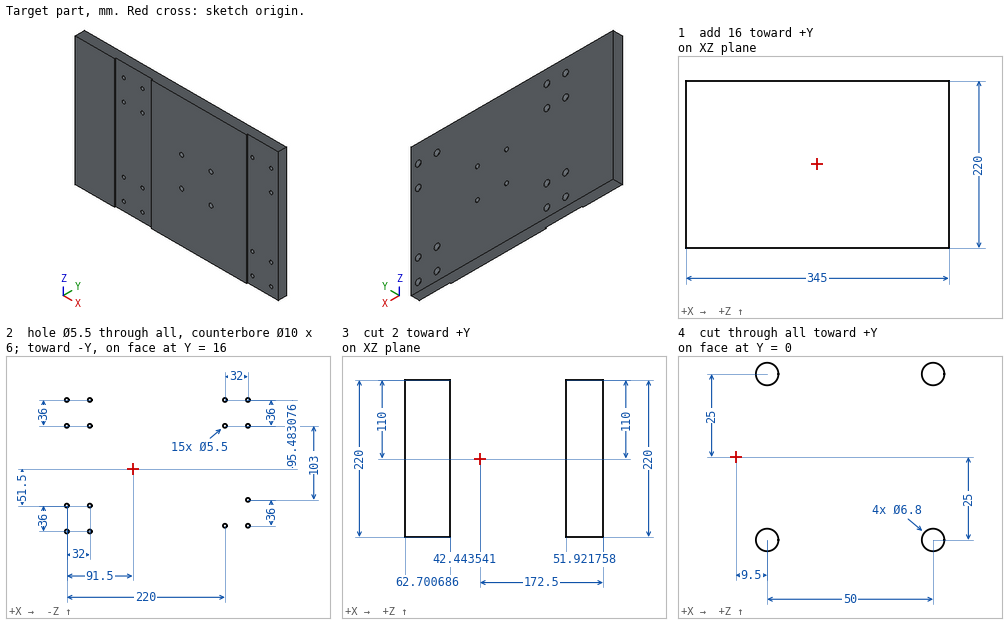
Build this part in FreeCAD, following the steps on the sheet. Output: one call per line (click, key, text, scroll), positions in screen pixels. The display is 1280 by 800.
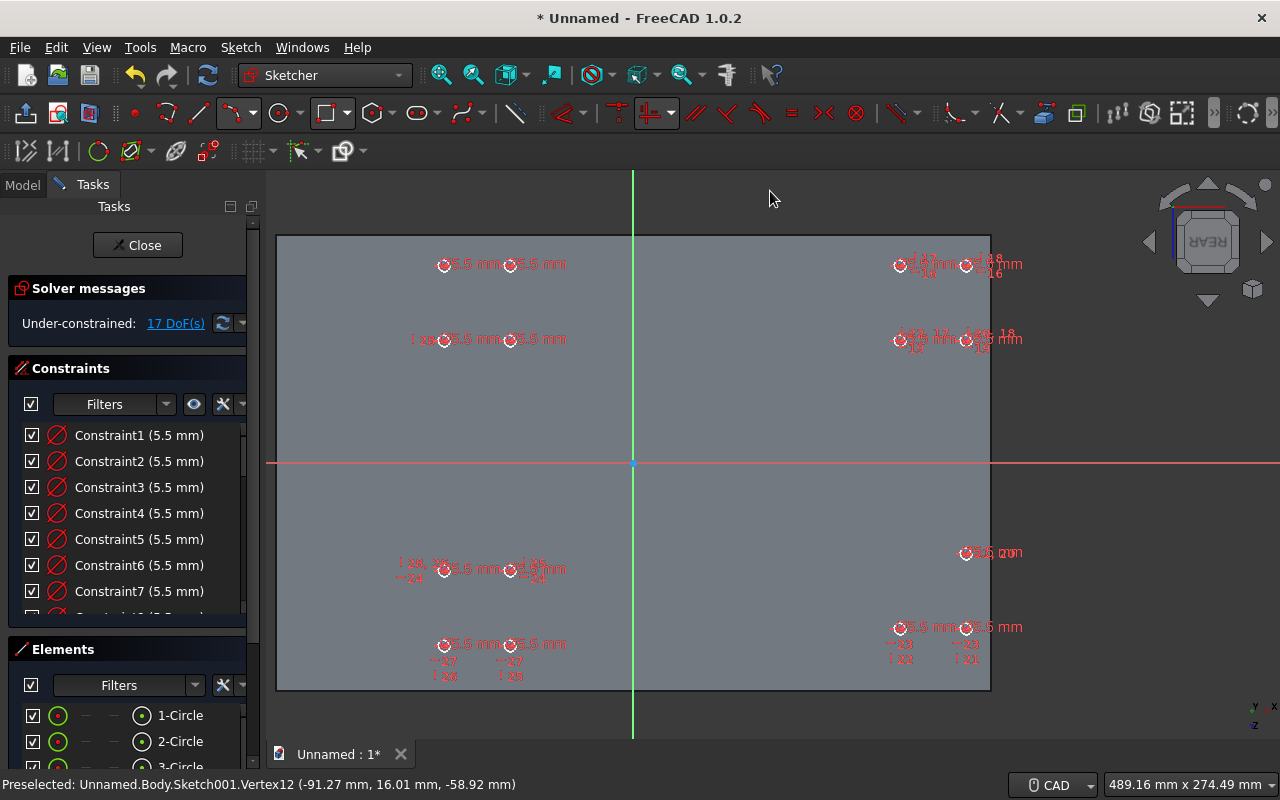
click(900, 341)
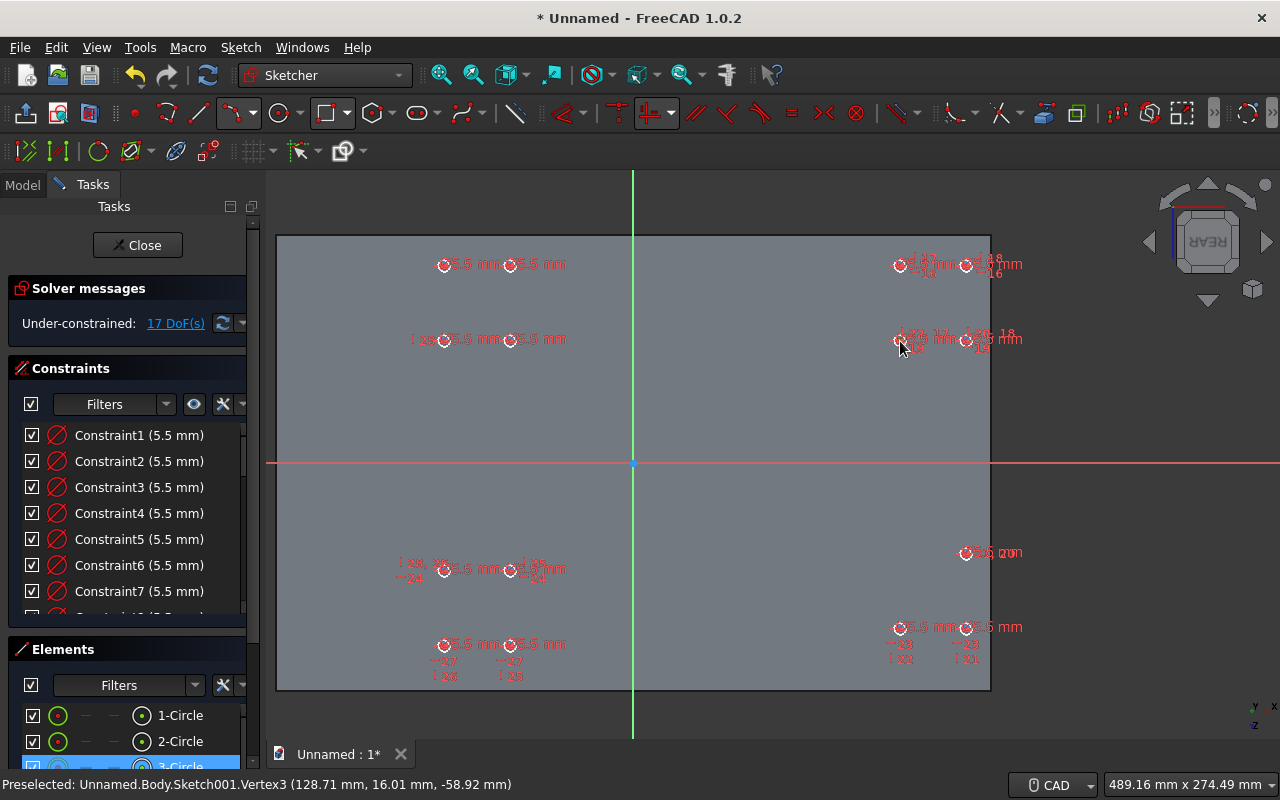
click(444, 341)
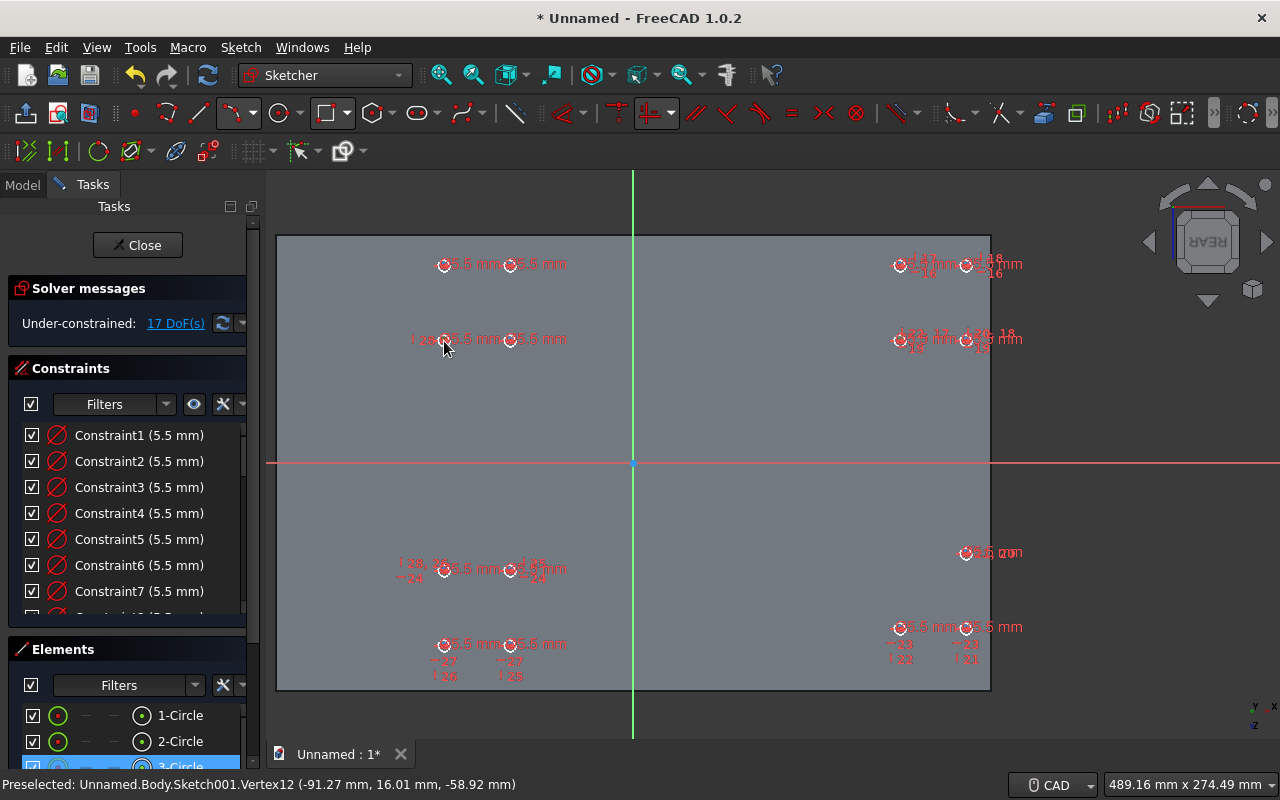
key(h)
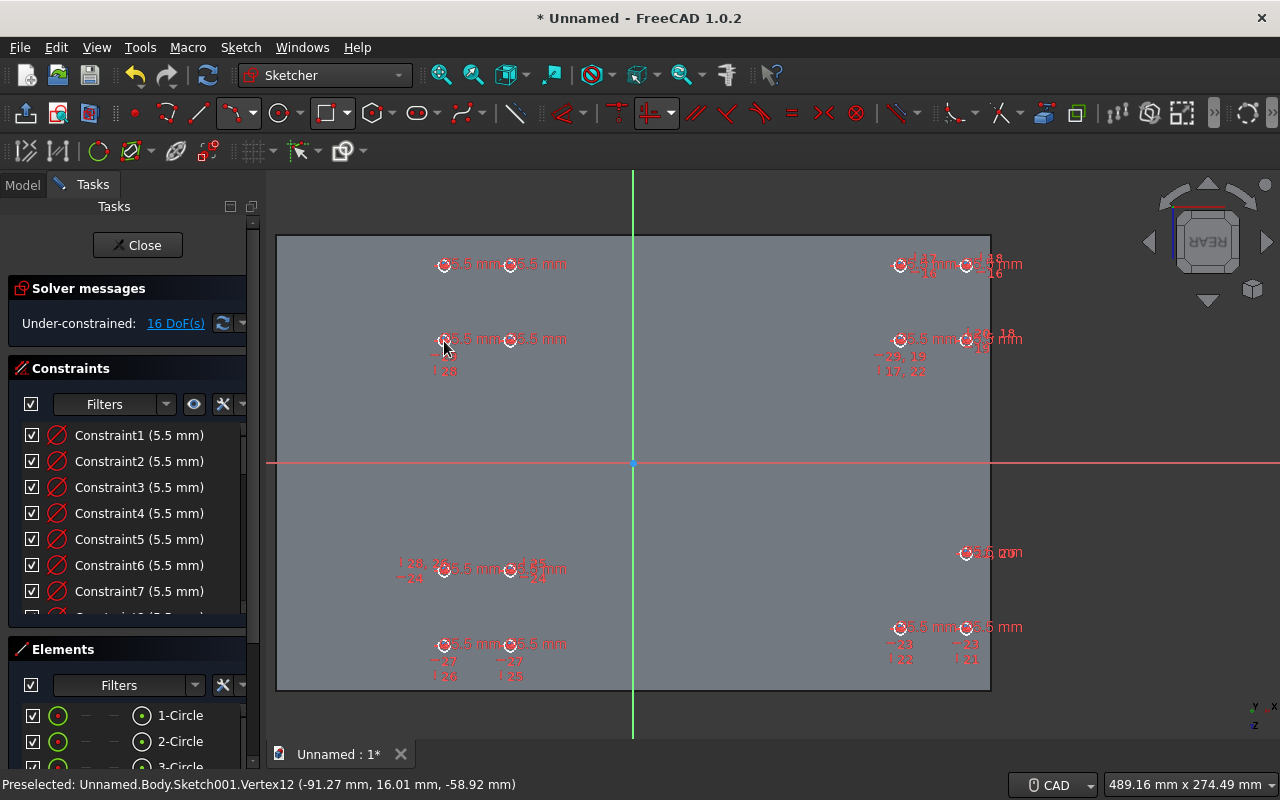
click(510, 571)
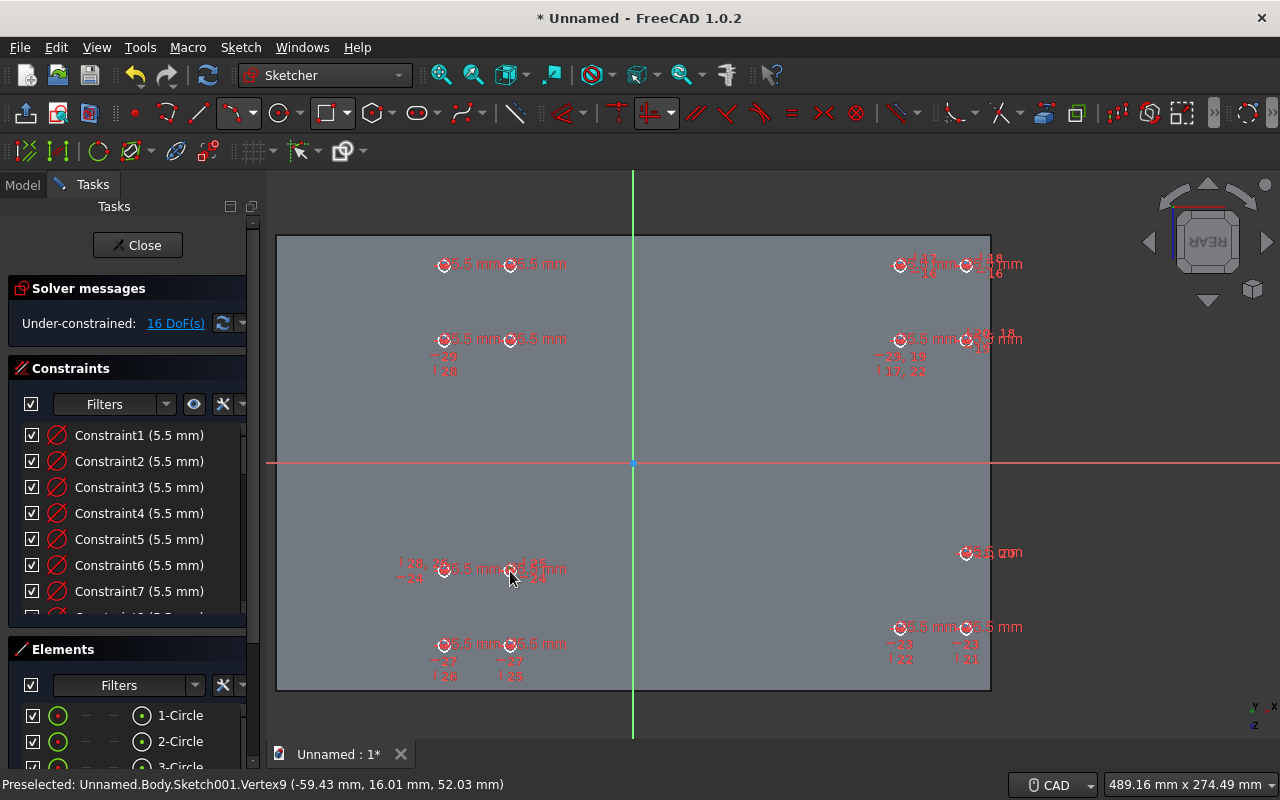
click(510, 341)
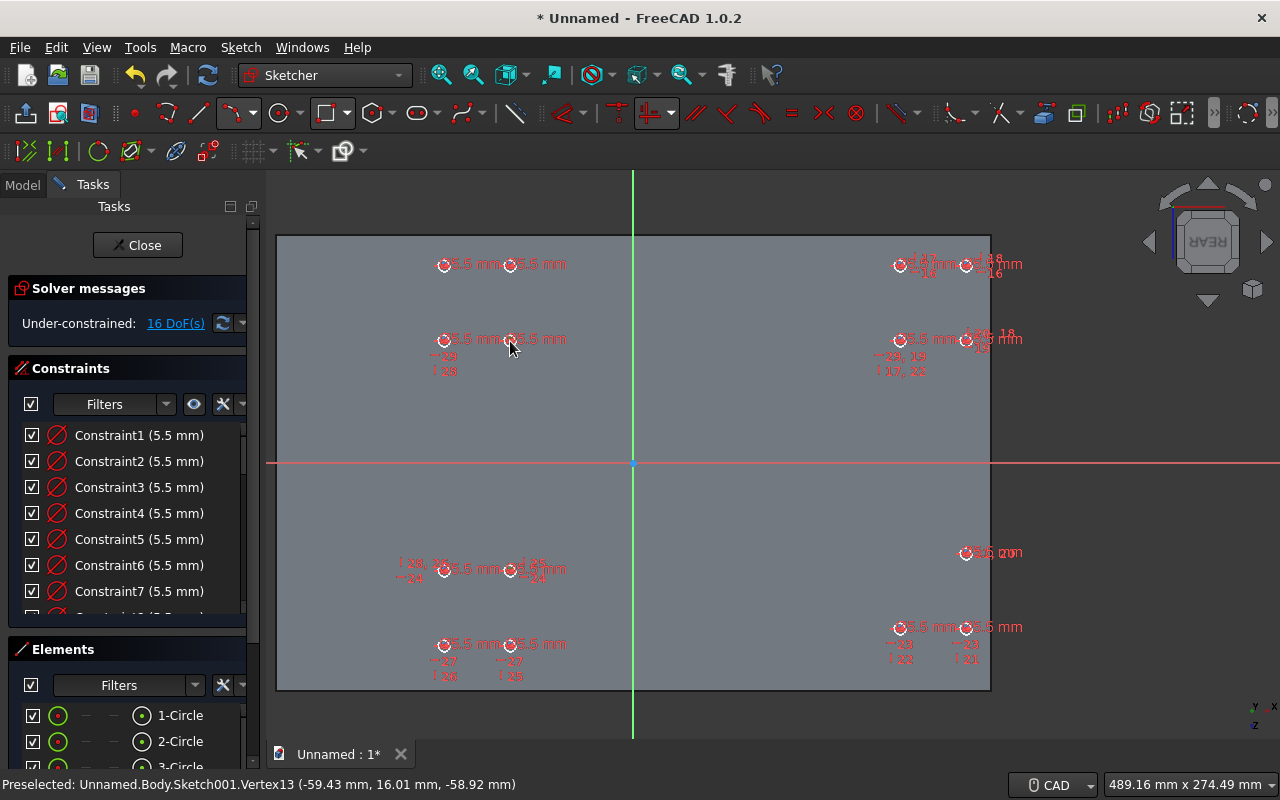
key(v)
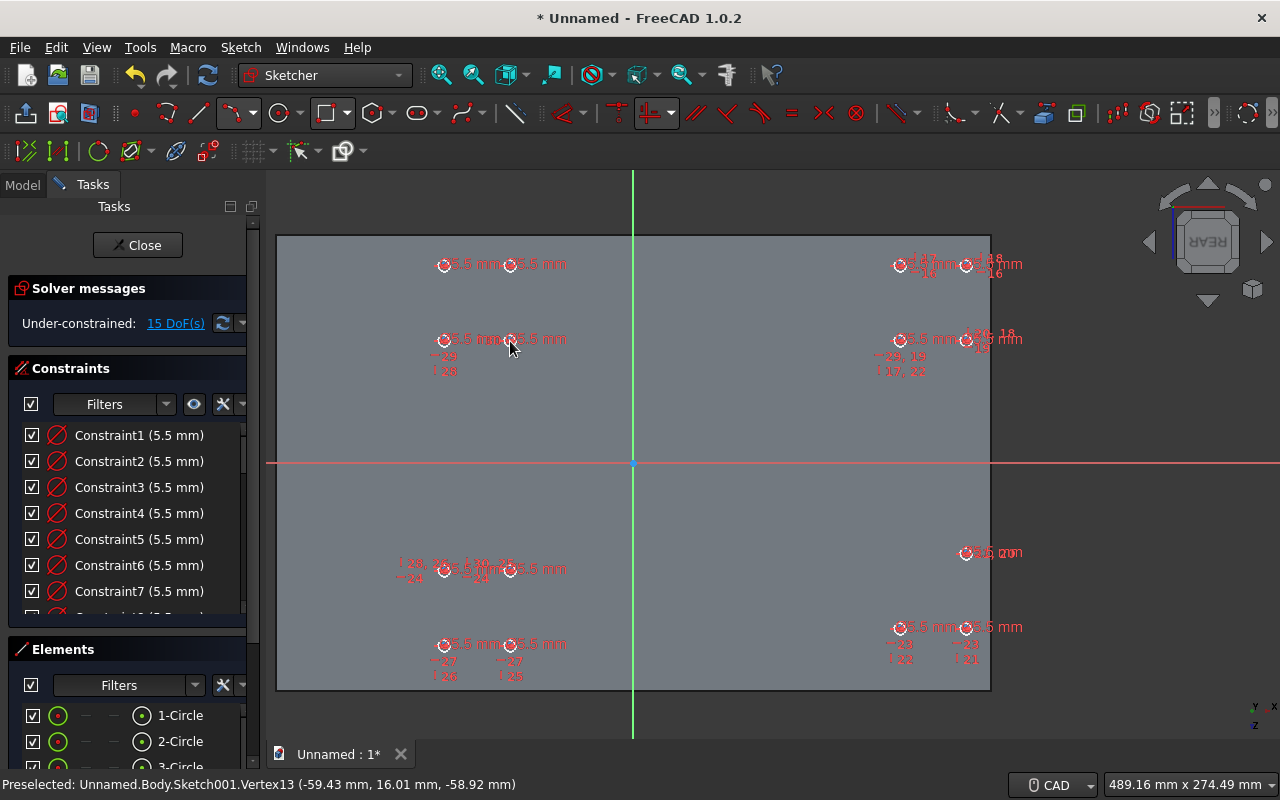
click(444, 341)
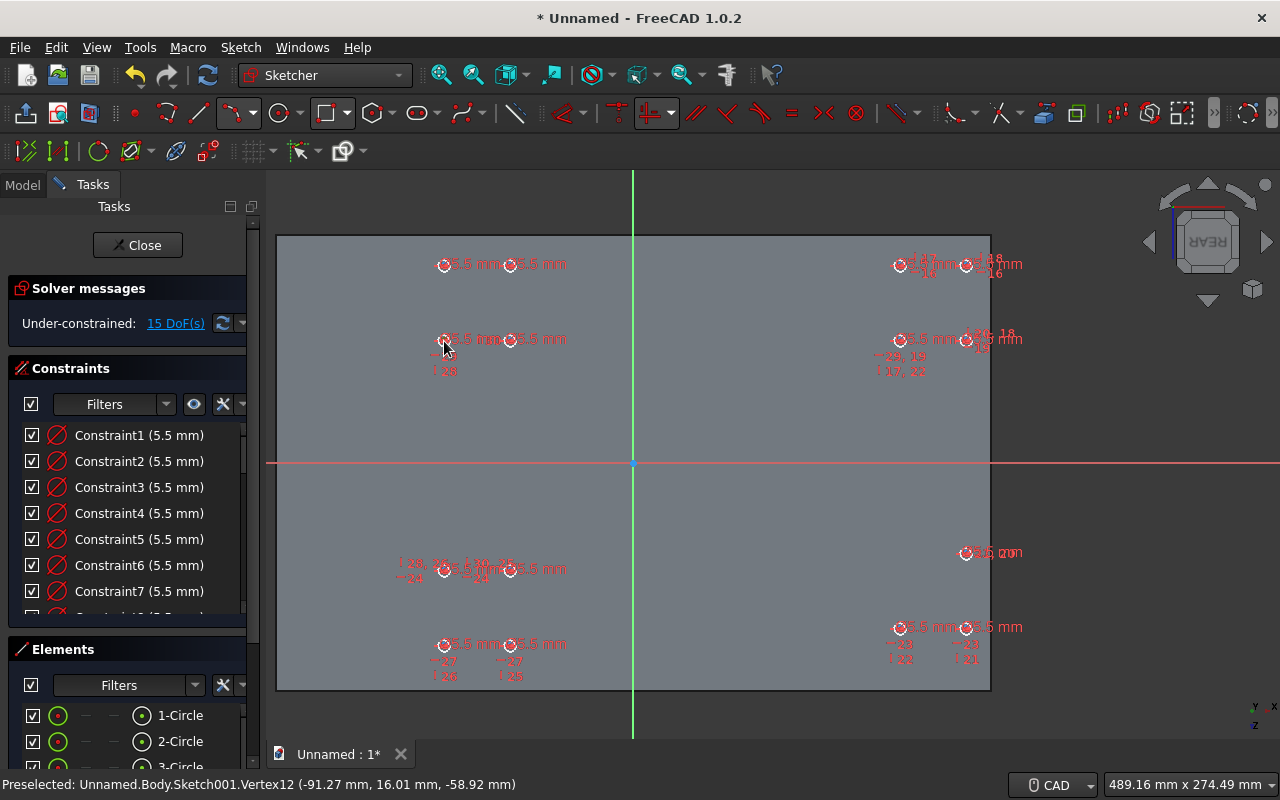
click(510, 341)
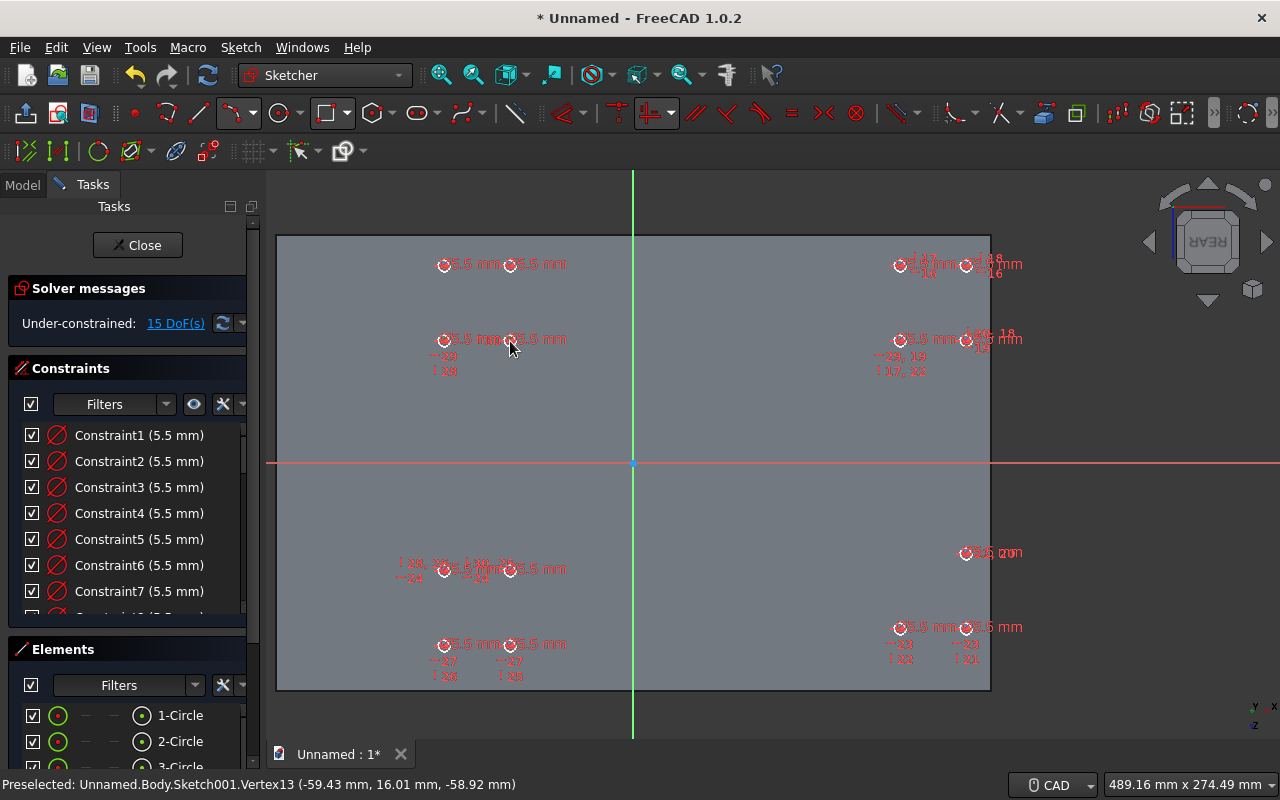
click(674, 114)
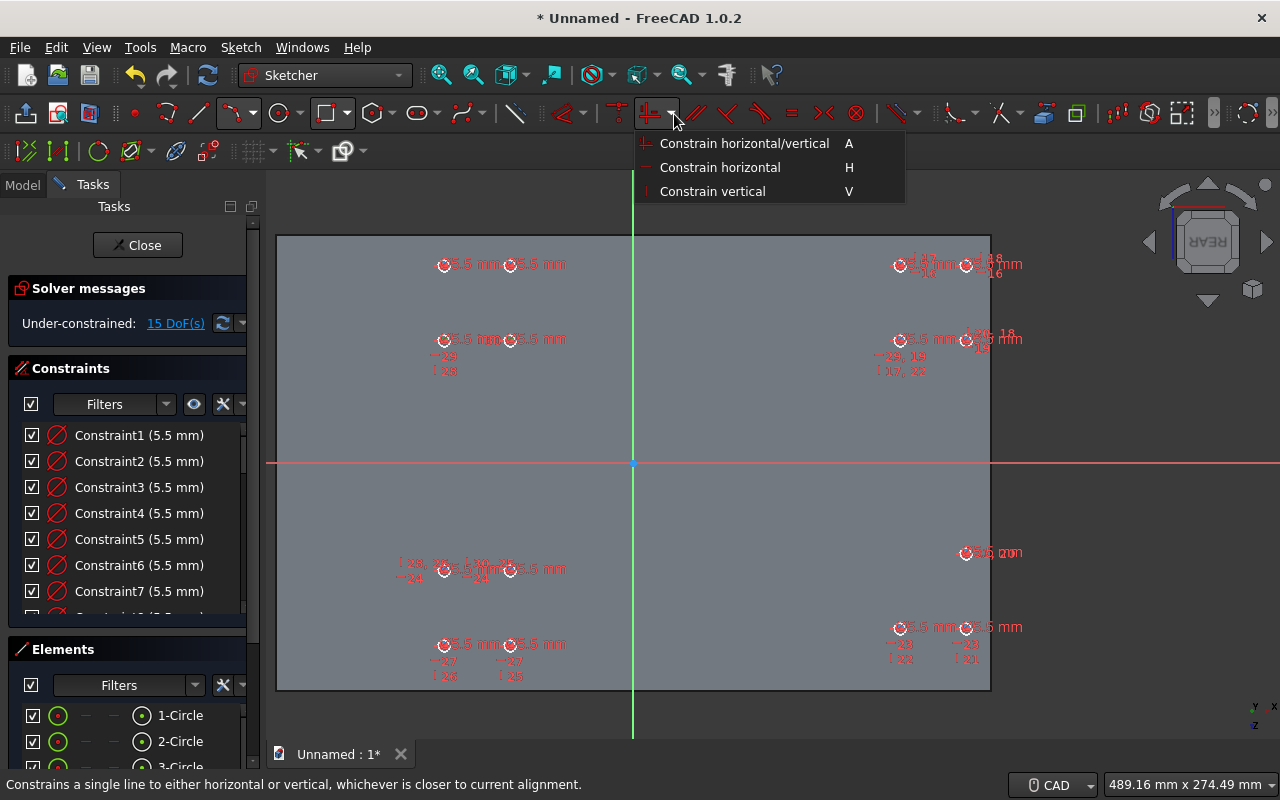
click(770, 167)